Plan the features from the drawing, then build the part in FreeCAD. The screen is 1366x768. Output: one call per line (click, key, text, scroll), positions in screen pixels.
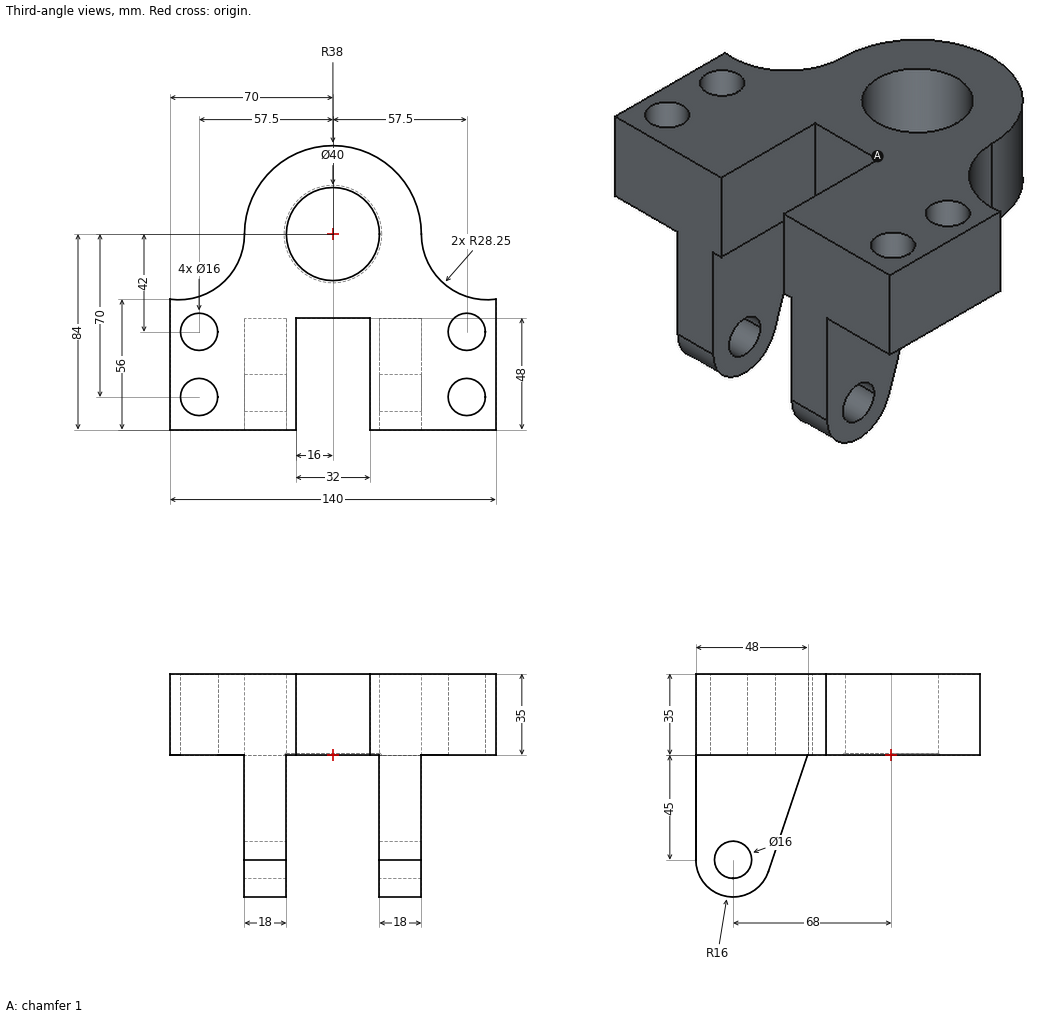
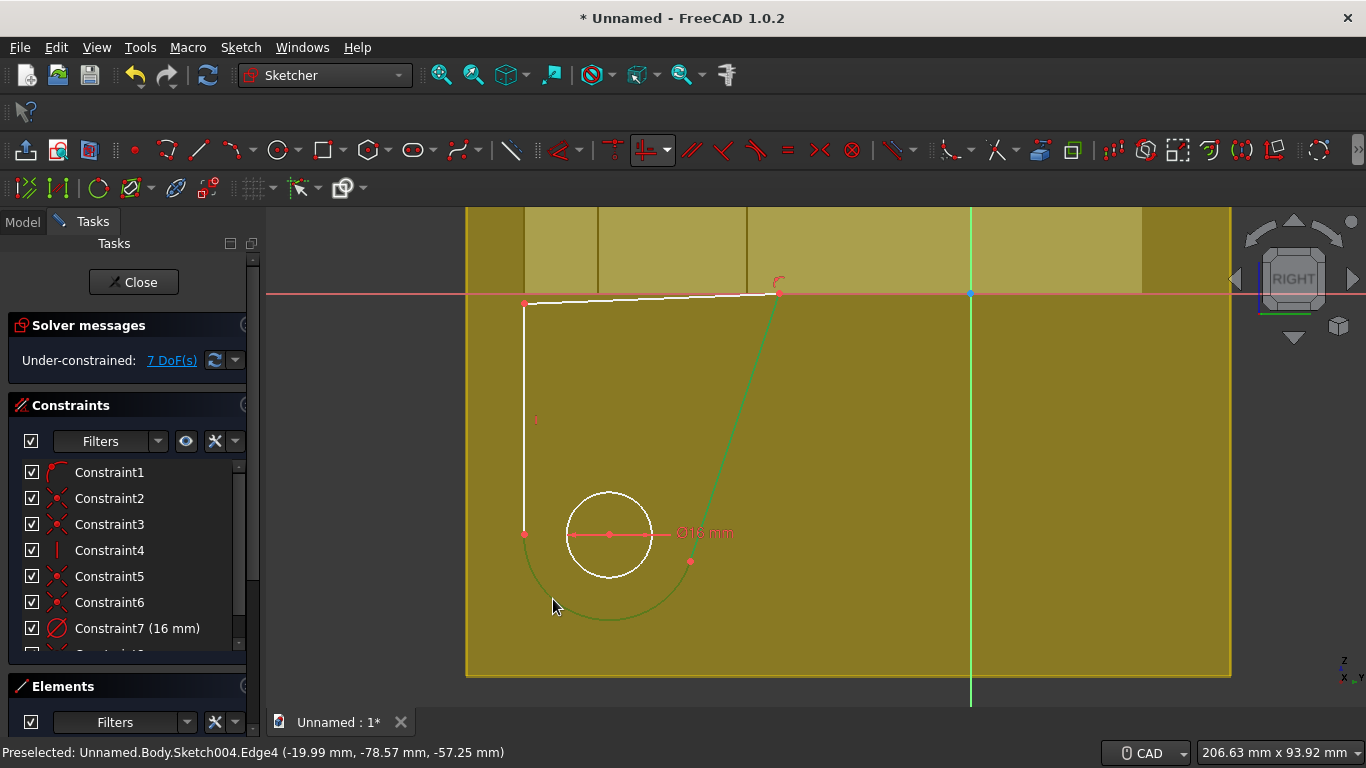
key(t)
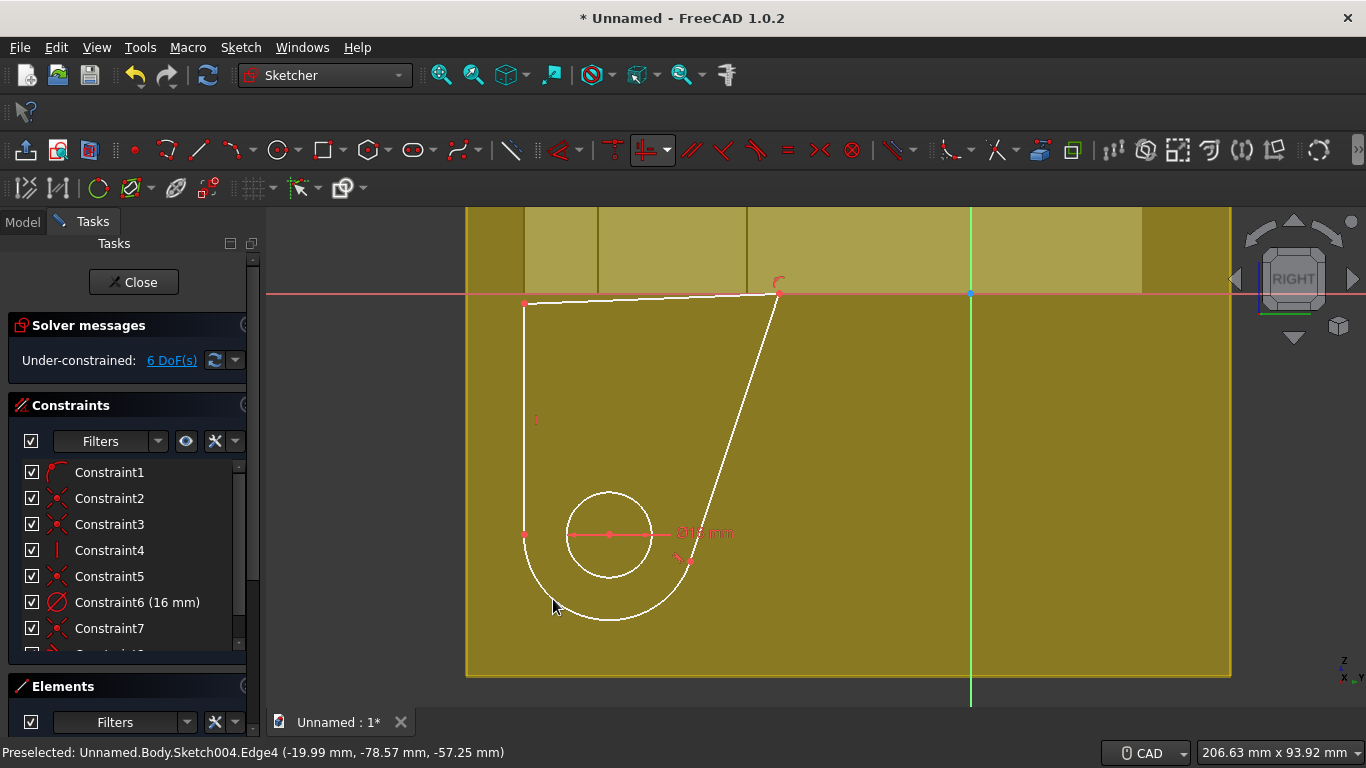
click(524, 373)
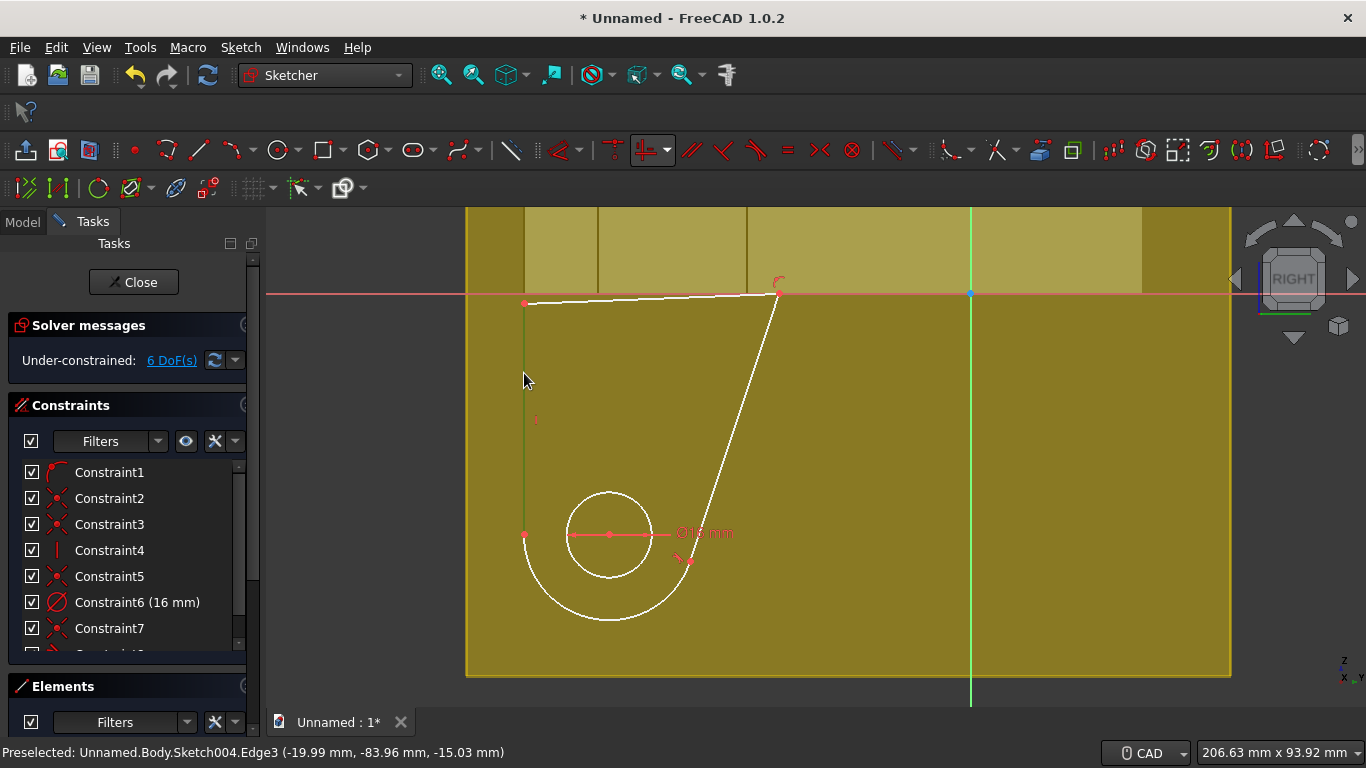
click(553, 599)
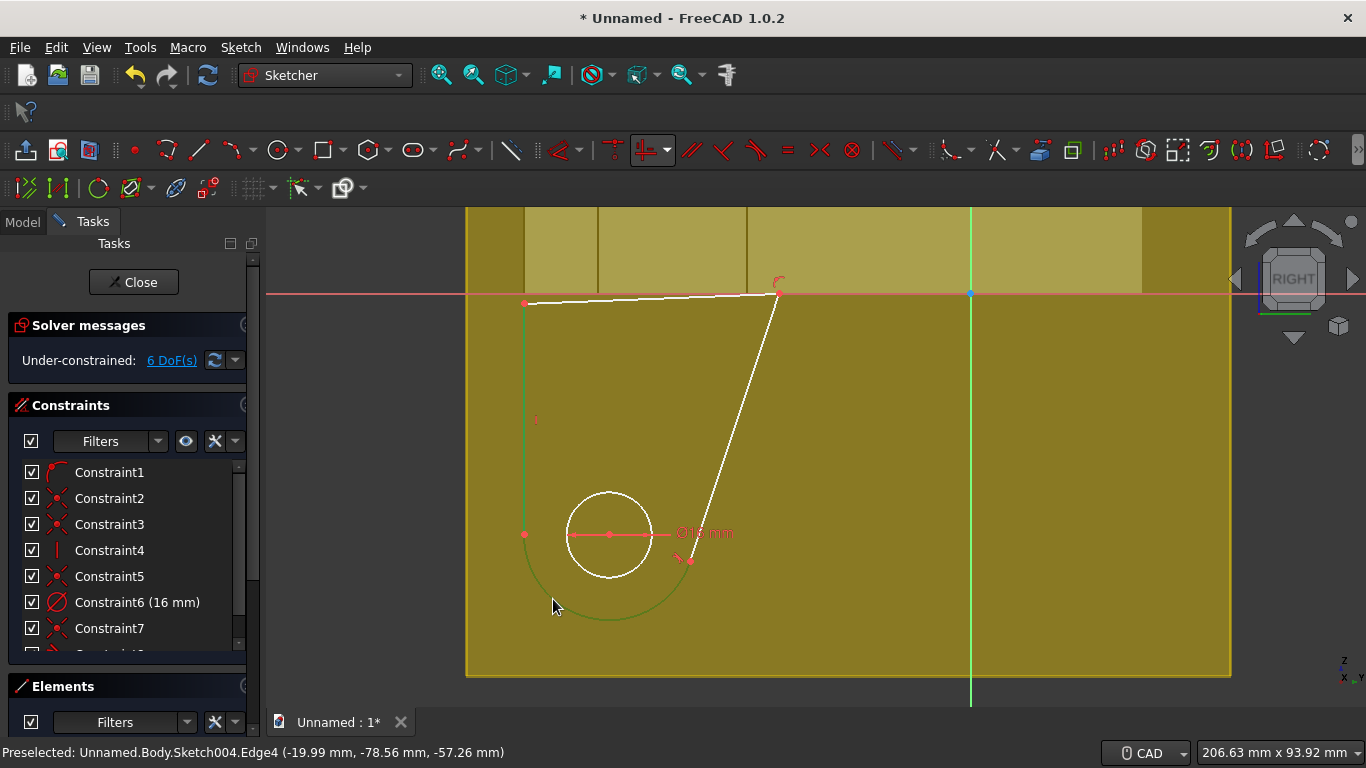
key(t)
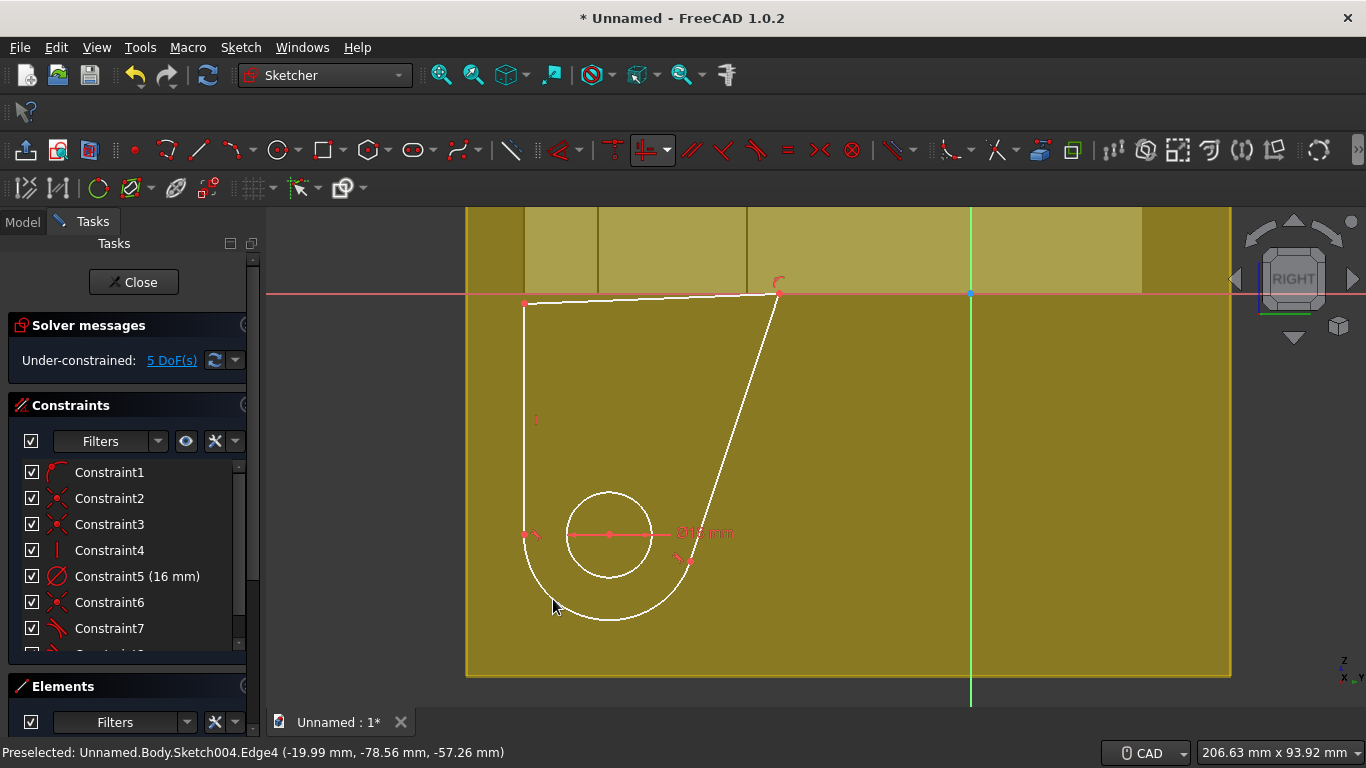
click(703, 297)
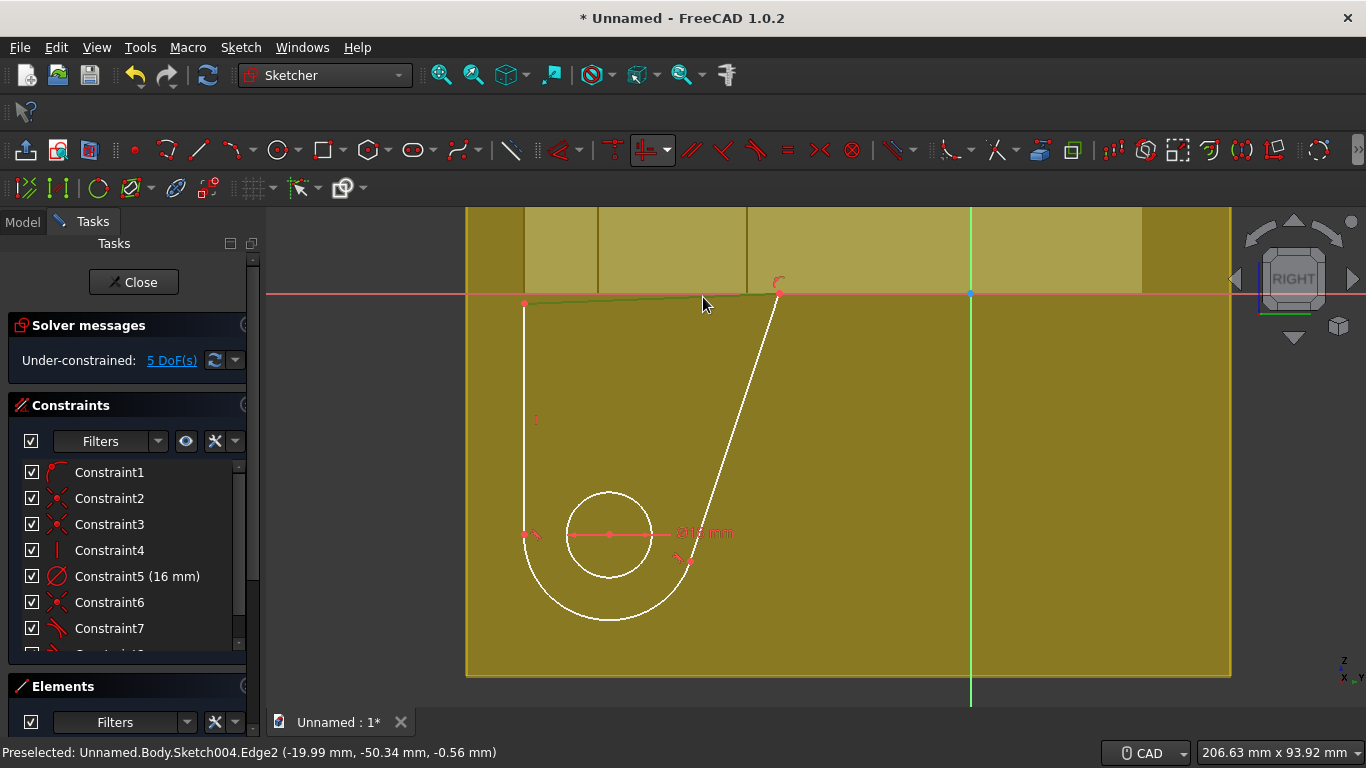
key(h)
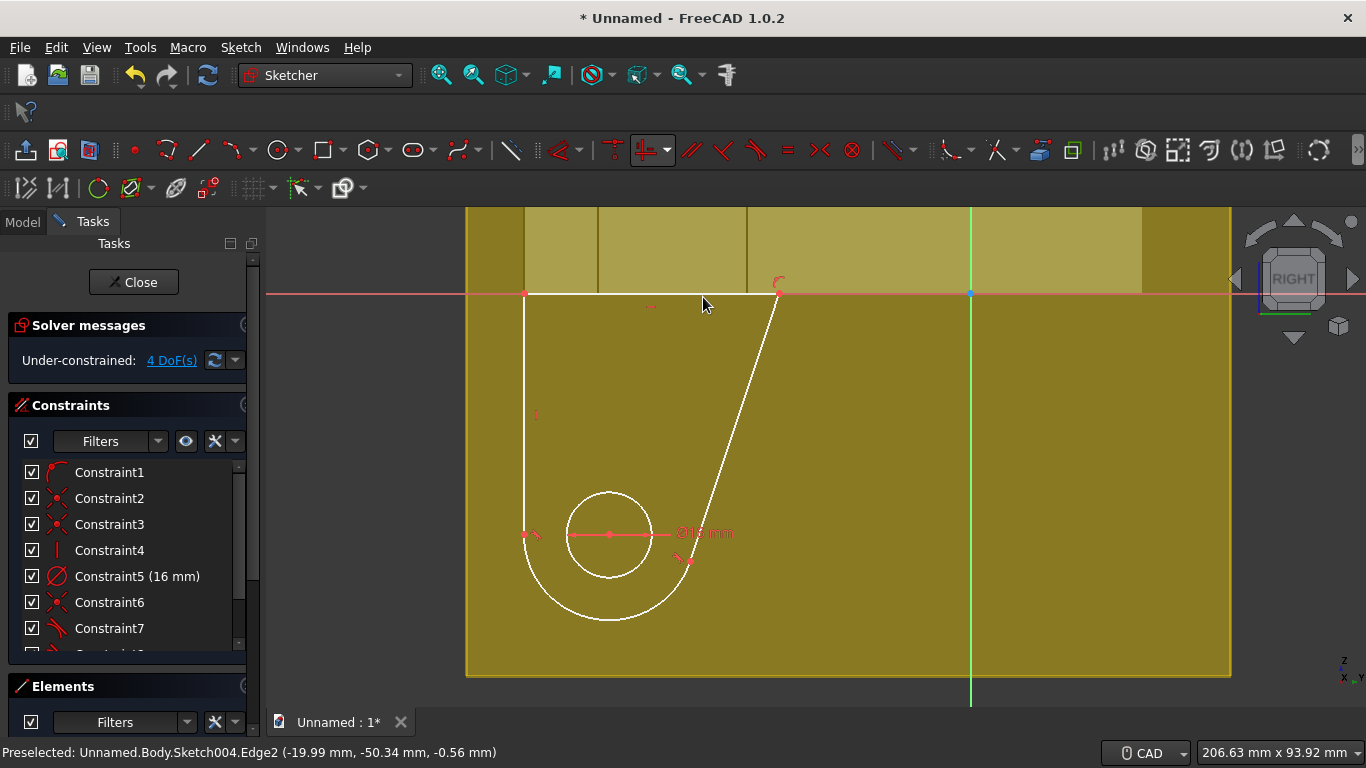
key(d)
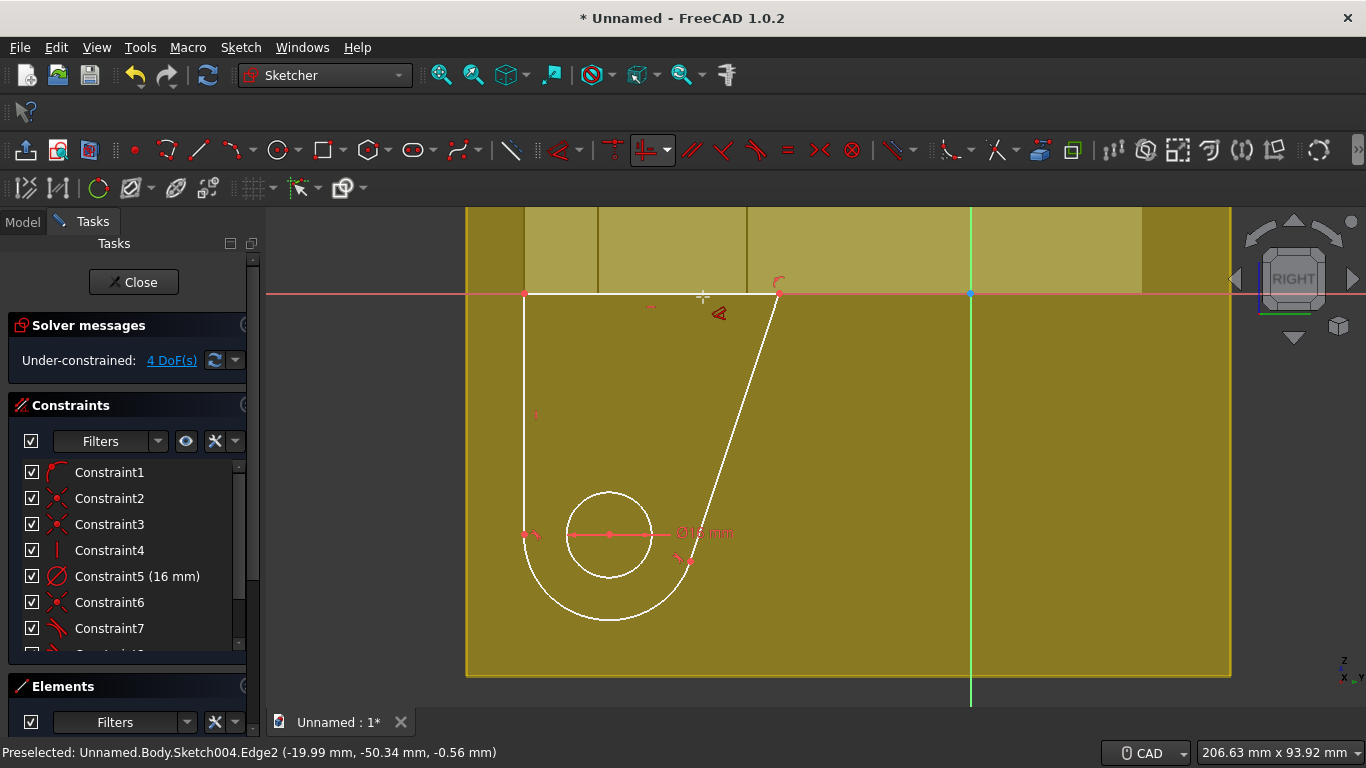
click(553, 599)
click(532, 623)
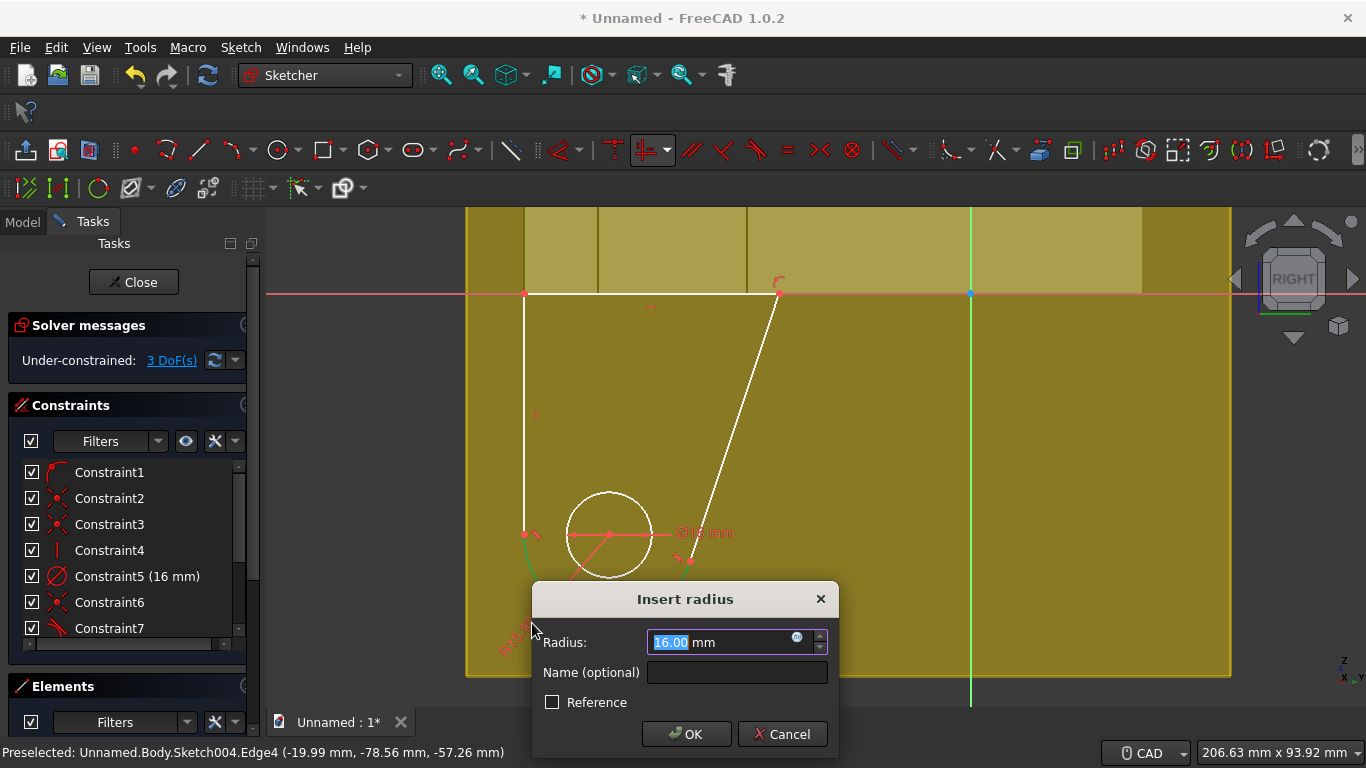
text(16)
key(Return)